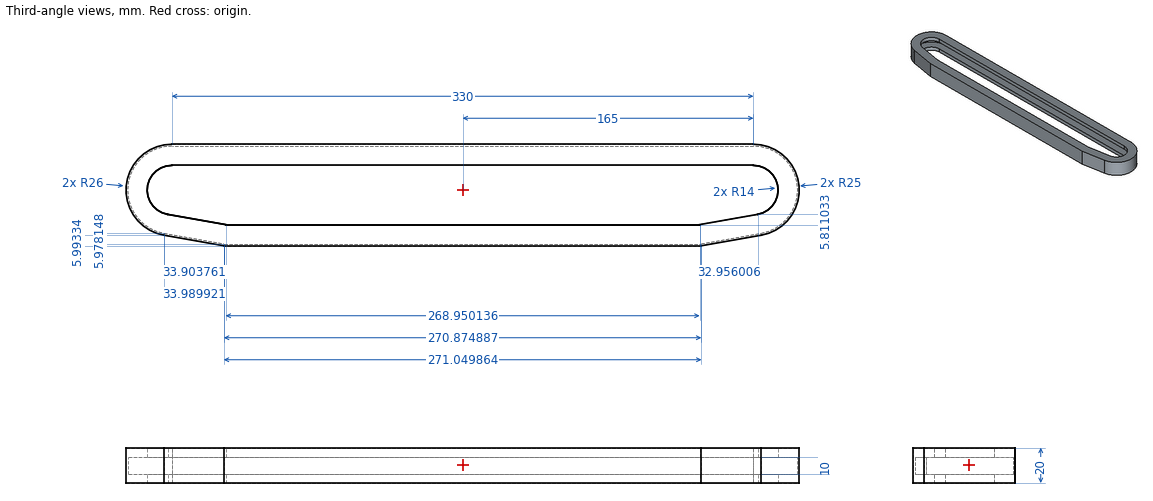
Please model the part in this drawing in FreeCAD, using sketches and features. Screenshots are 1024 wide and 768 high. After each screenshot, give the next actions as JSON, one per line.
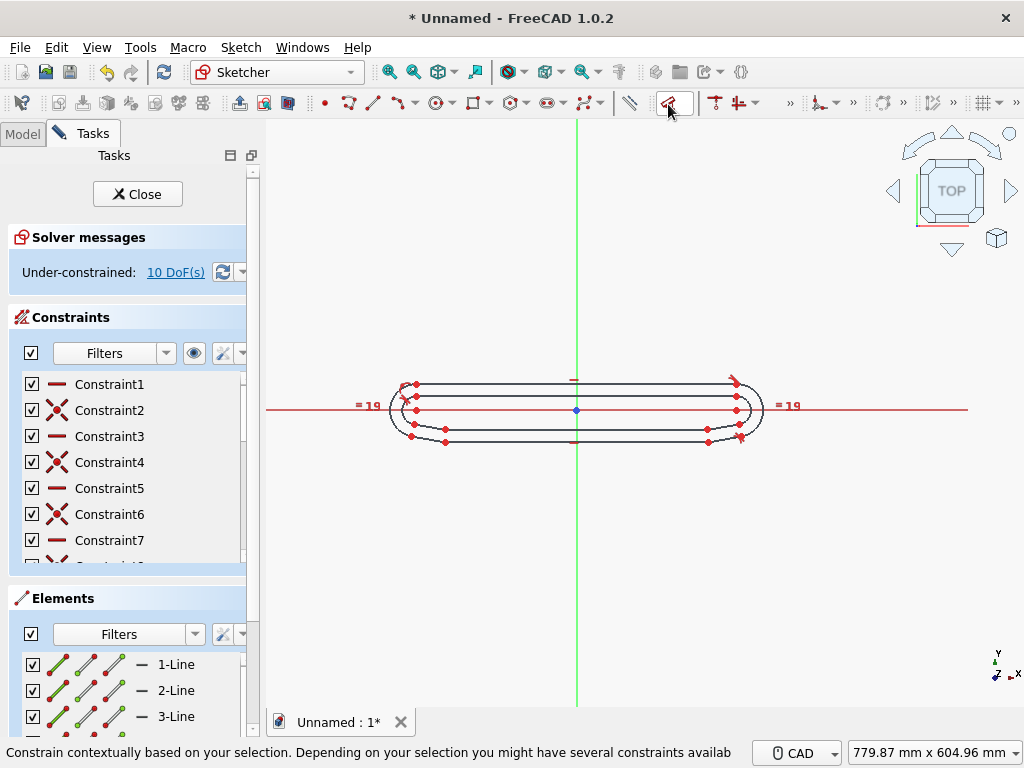
{"action": "scroll", "coordinate": [396, 394], "scroll_direction": "up", "scroll_amount": 3}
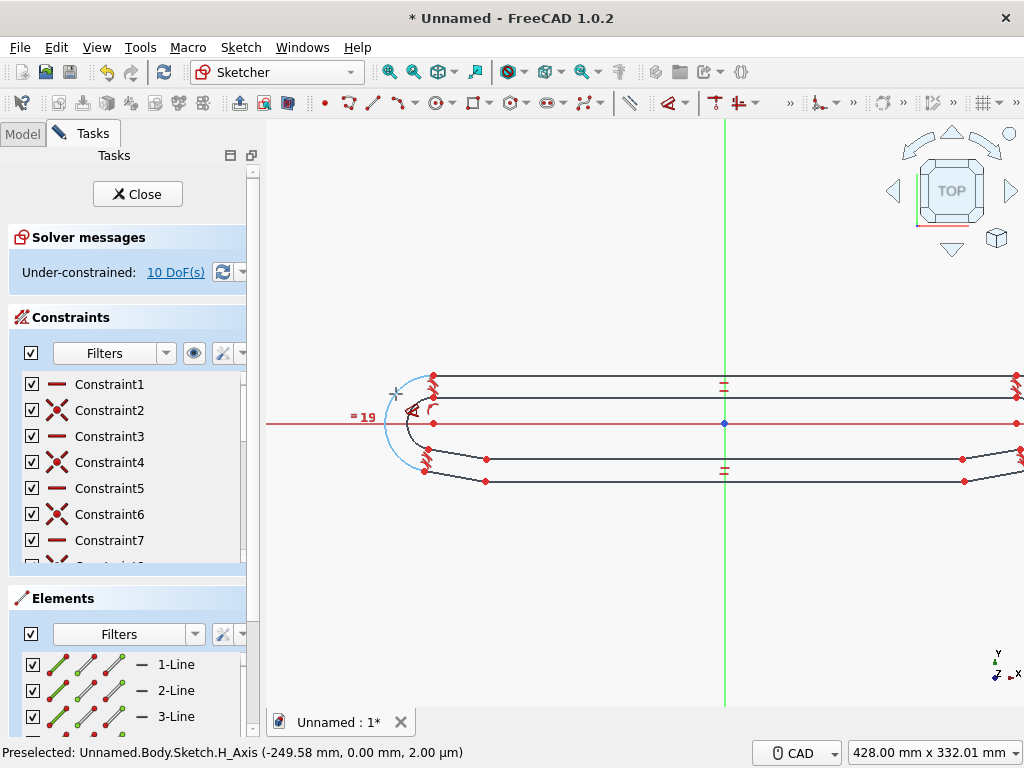
{"action": "left_click", "coordinate": [396, 393]}
{"action": "left_click", "coordinate": [371, 373]}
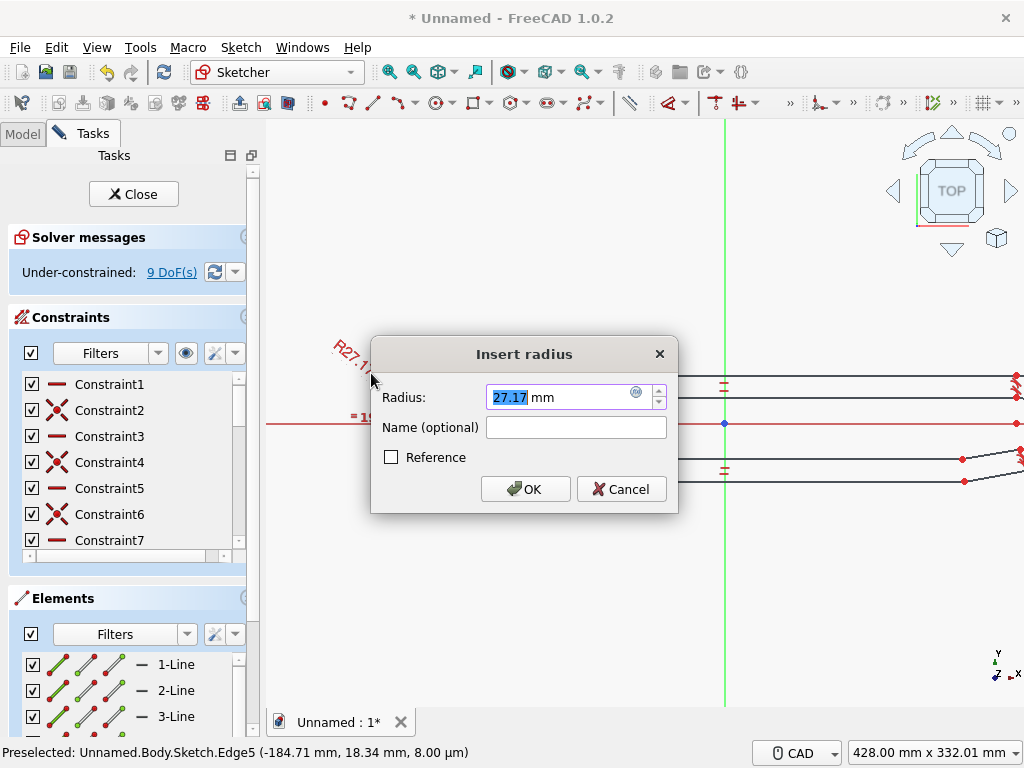
{"action": "type", "text": "26"}
{"action": "key", "text": "Return"}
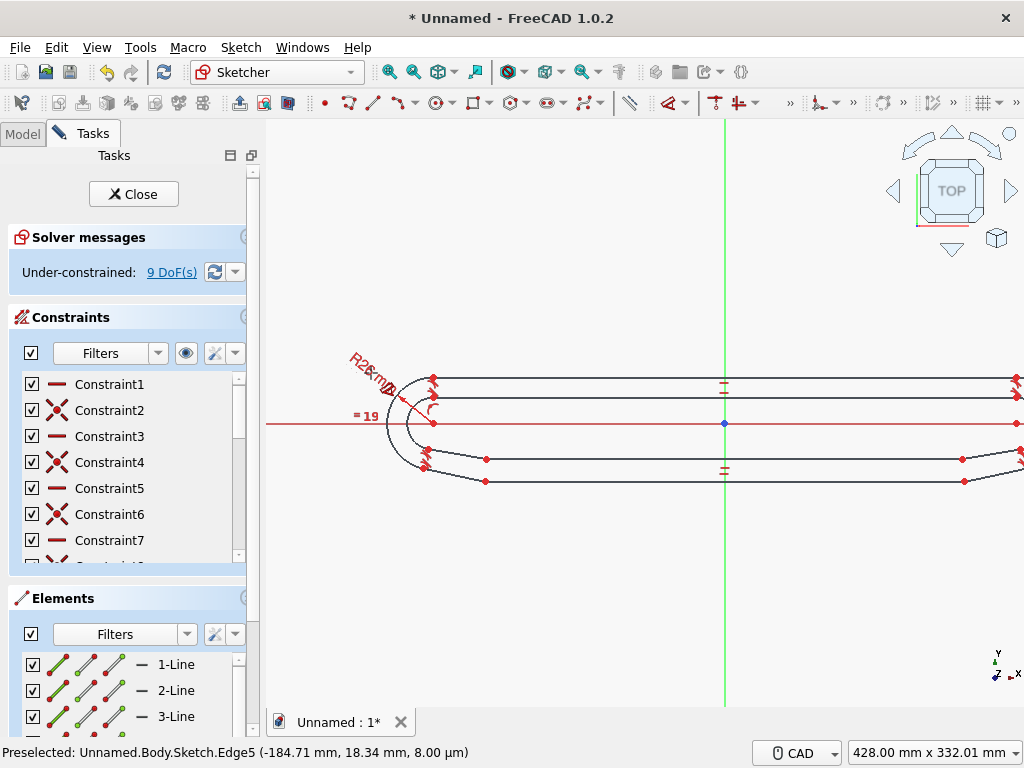
{"action": "scroll", "coordinate": [396, 394], "scroll_direction": "down", "scroll_amount": 3}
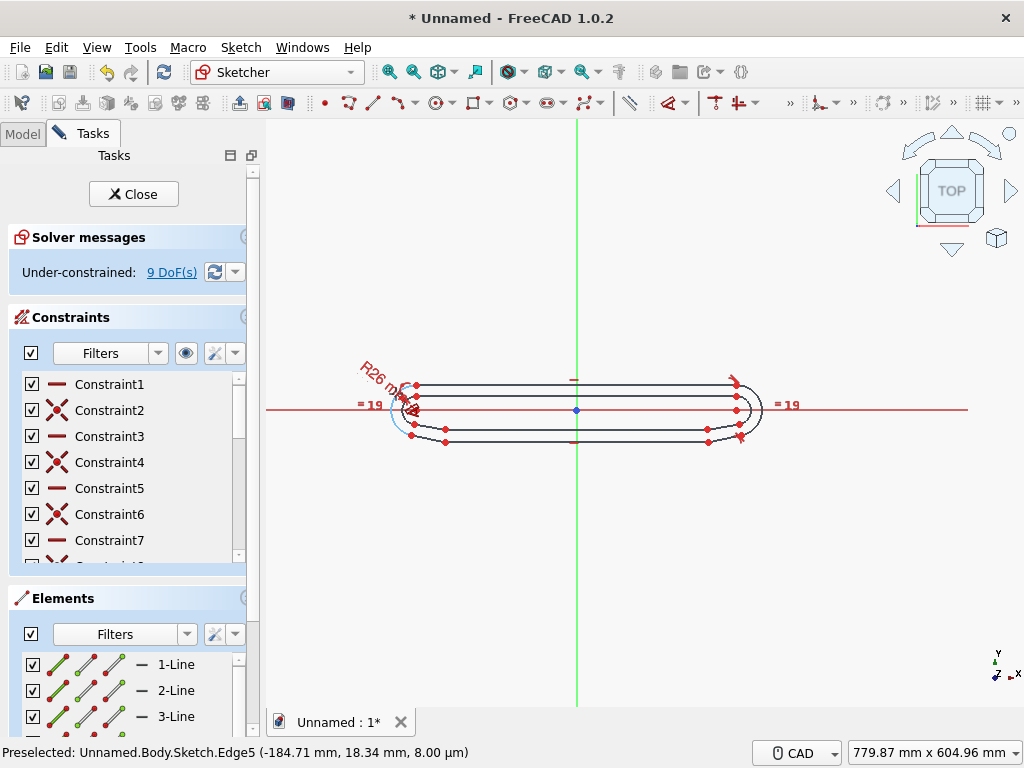
{"action": "scroll", "coordinate": [749, 417], "scroll_direction": "up", "scroll_amount": 6}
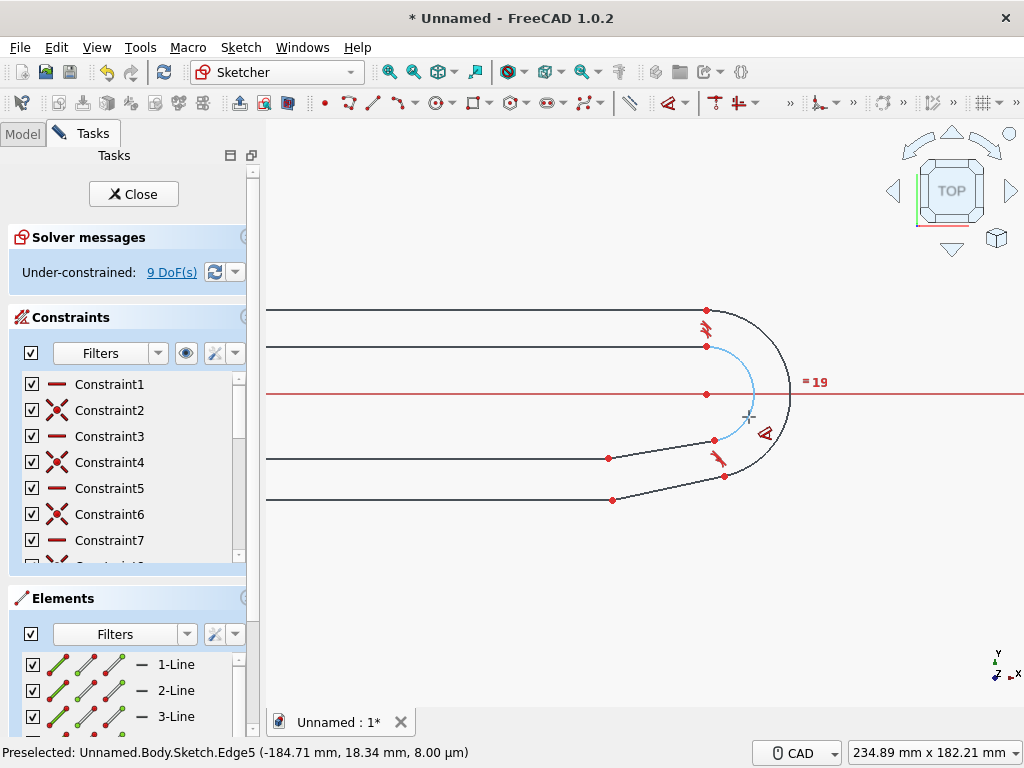
{"action": "left_click", "coordinate": [748, 417]}
{"action": "left_click", "coordinate": [668, 464]}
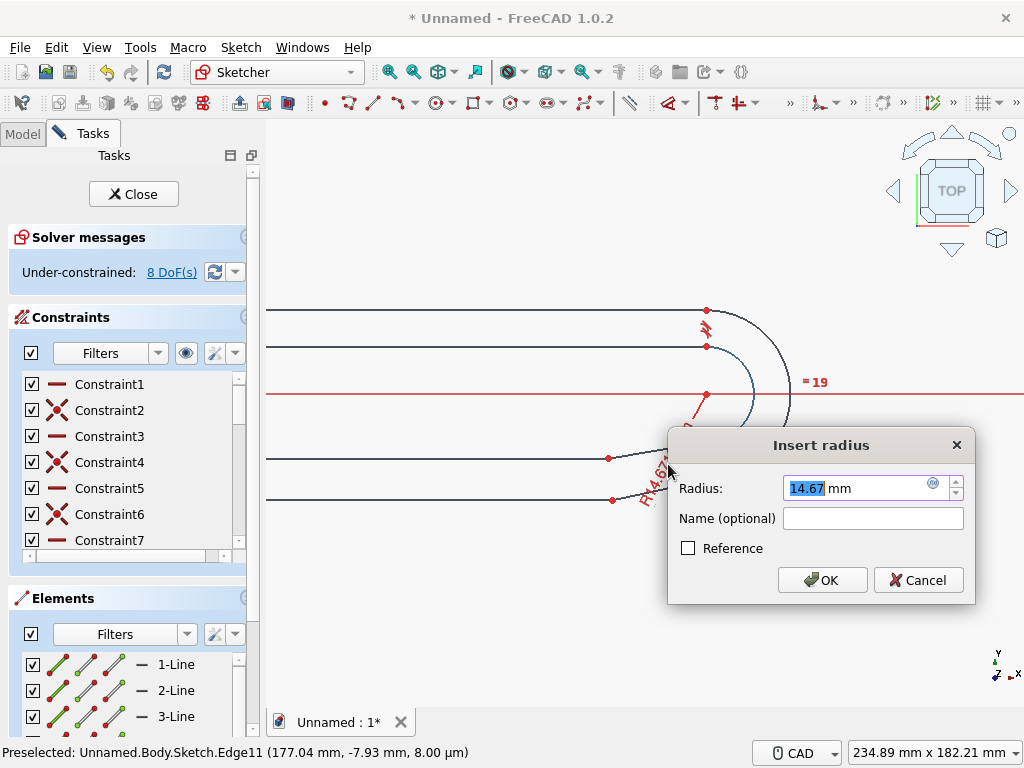
{"action": "type", "text": "14"}
{"action": "key", "text": "Return"}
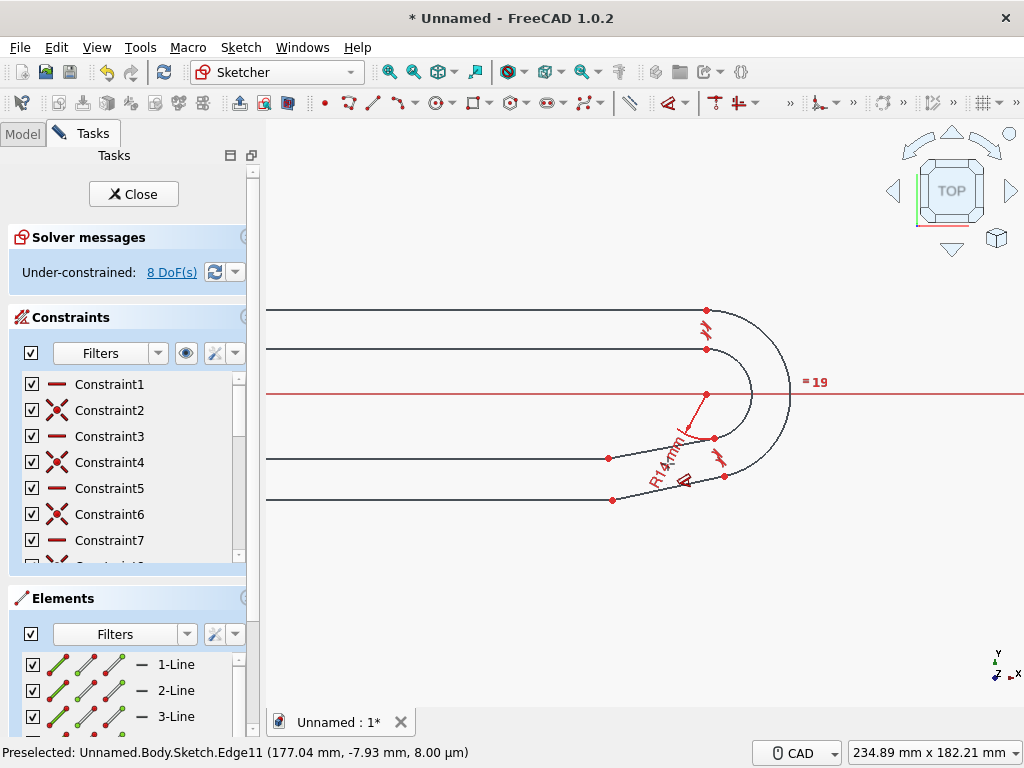
{"action": "left_click", "coordinate": [388, 310]}
{"action": "left_click", "coordinate": [500, 276]}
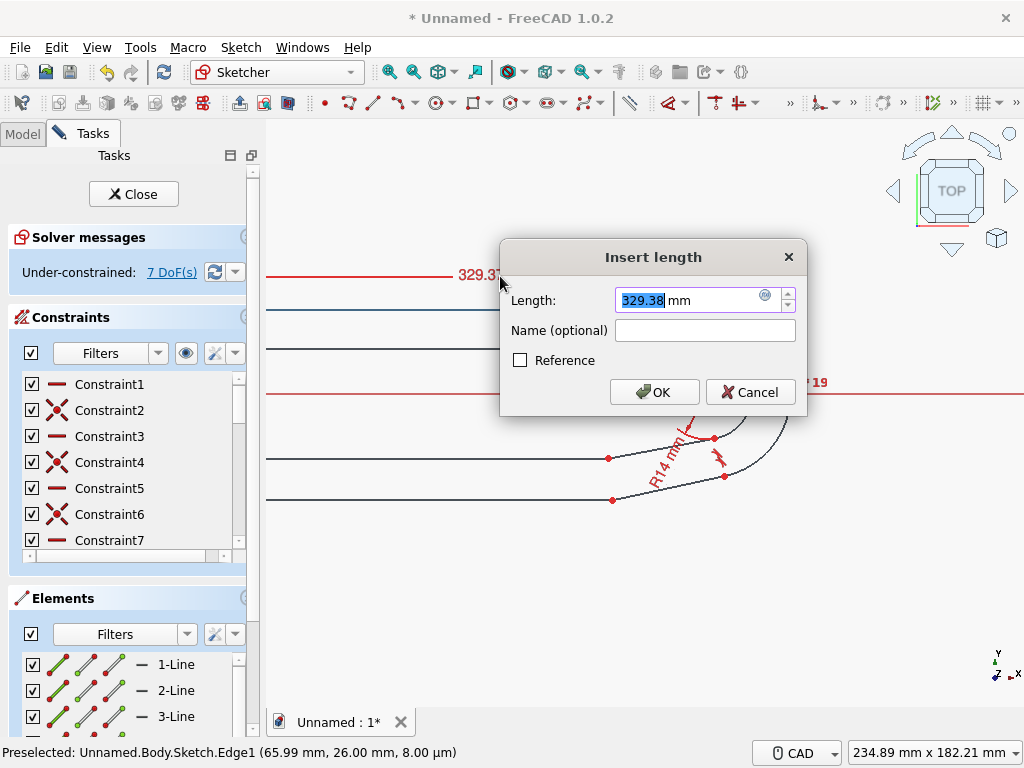
{"action": "type", "text": "330"}
{"action": "key", "text": "Return"}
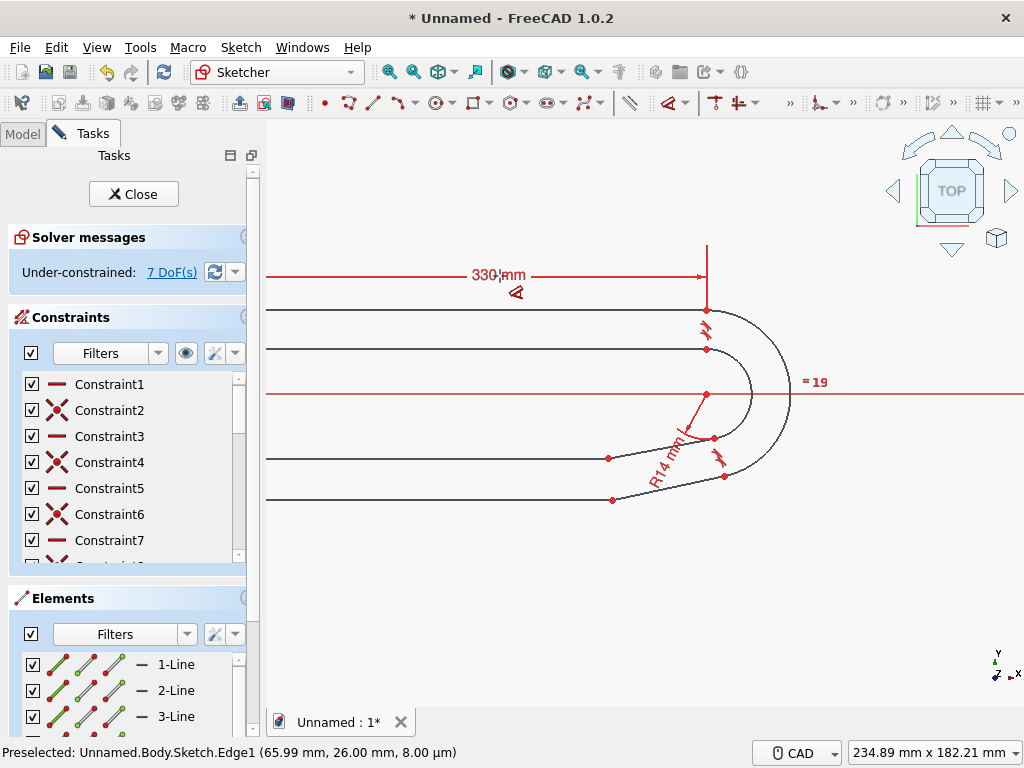
{"action": "left_click", "coordinate": [707, 310]}
{"action": "left_click", "coordinate": [405, 276]}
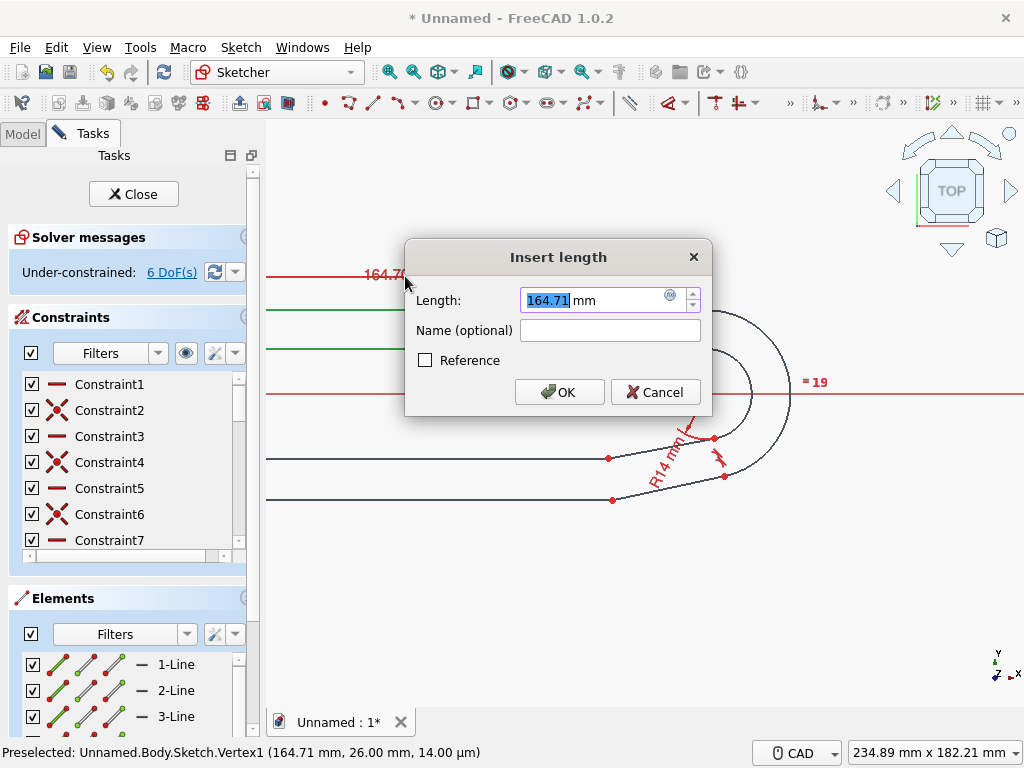
{"action": "type", "text": "165"}
{"action": "key", "text": "Return"}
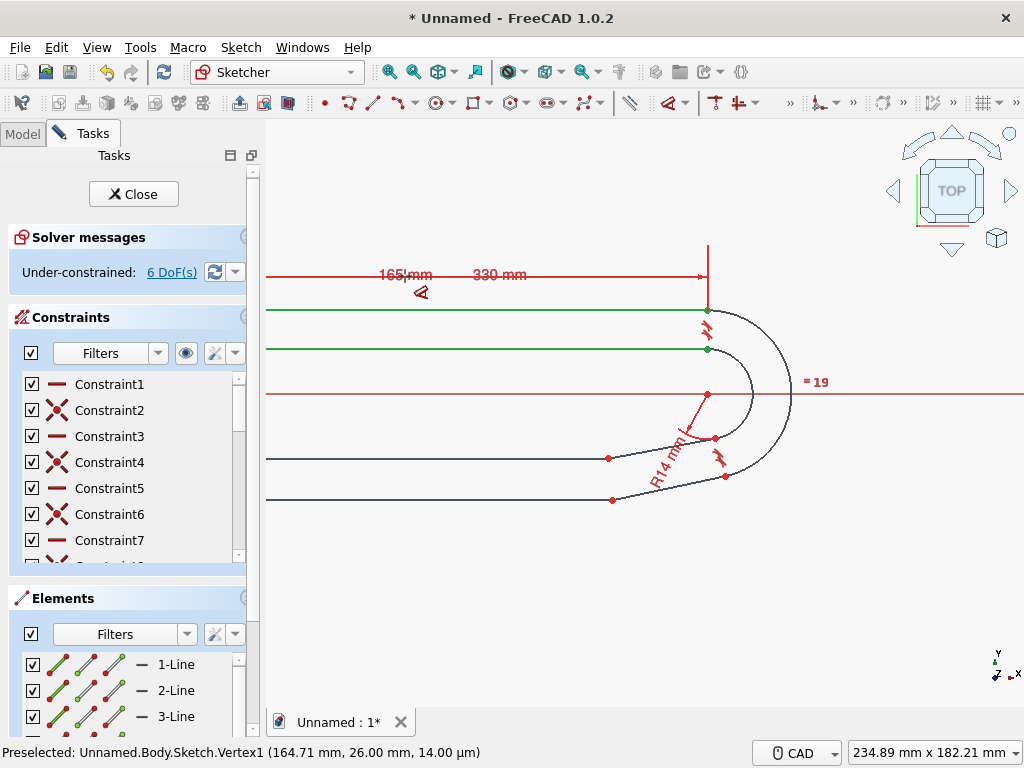
{"action": "scroll", "coordinate": [750, 417], "scroll_direction": "down", "scroll_amount": 6}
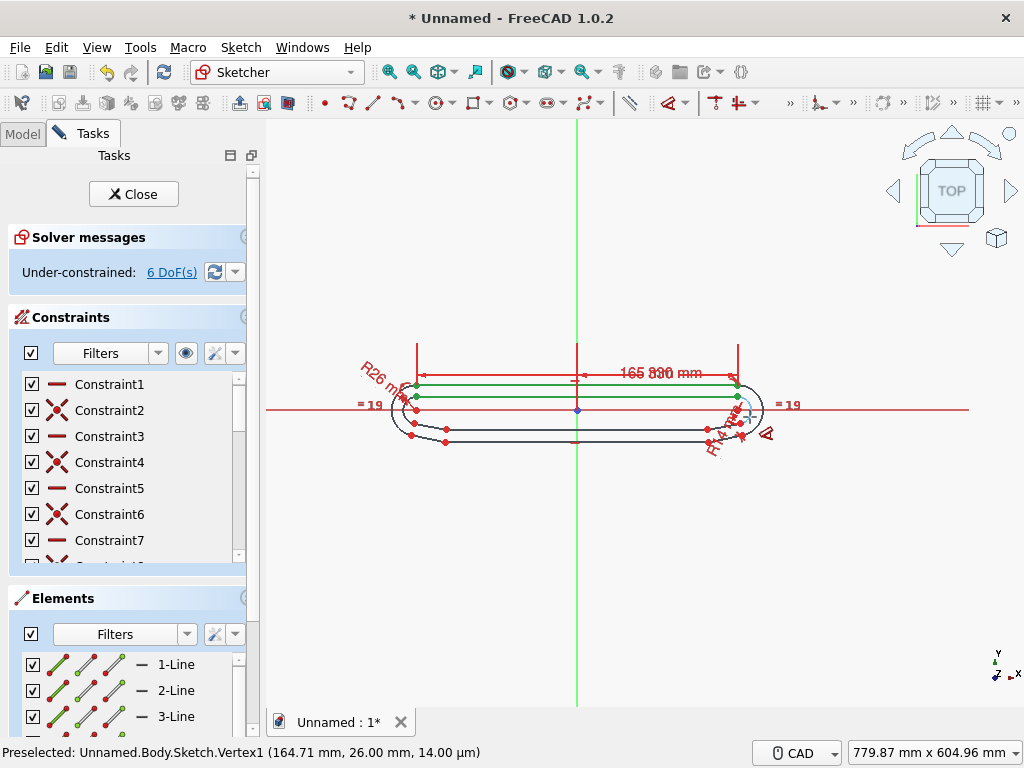
{"action": "scroll", "coordinate": [422, 437], "scroll_direction": "up", "scroll_amount": 10}